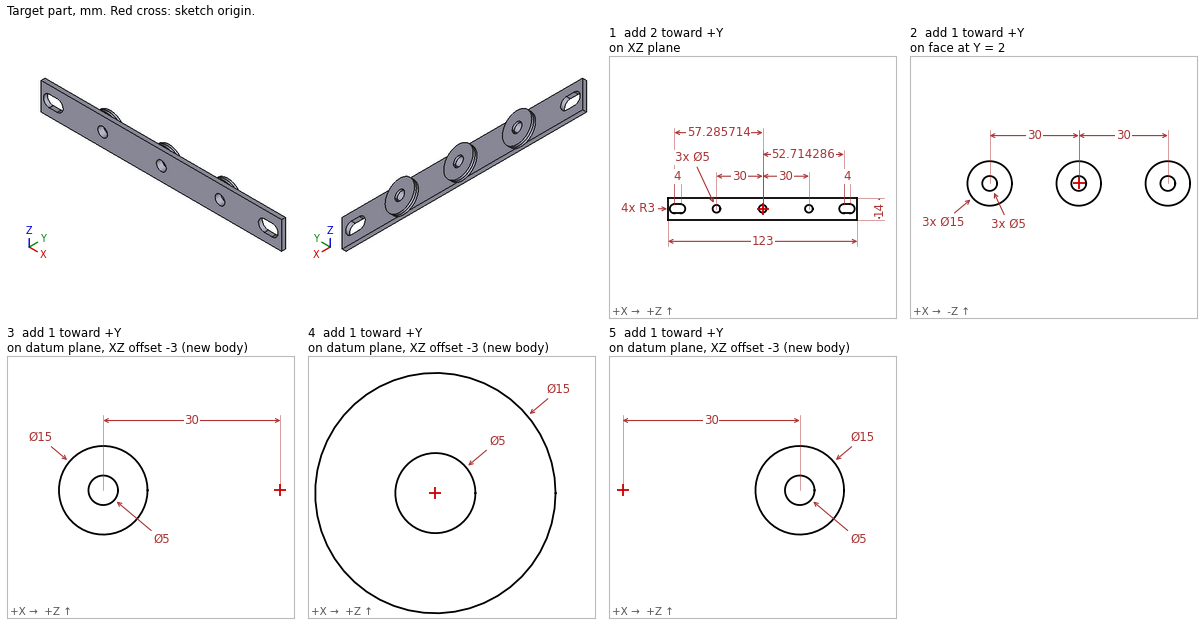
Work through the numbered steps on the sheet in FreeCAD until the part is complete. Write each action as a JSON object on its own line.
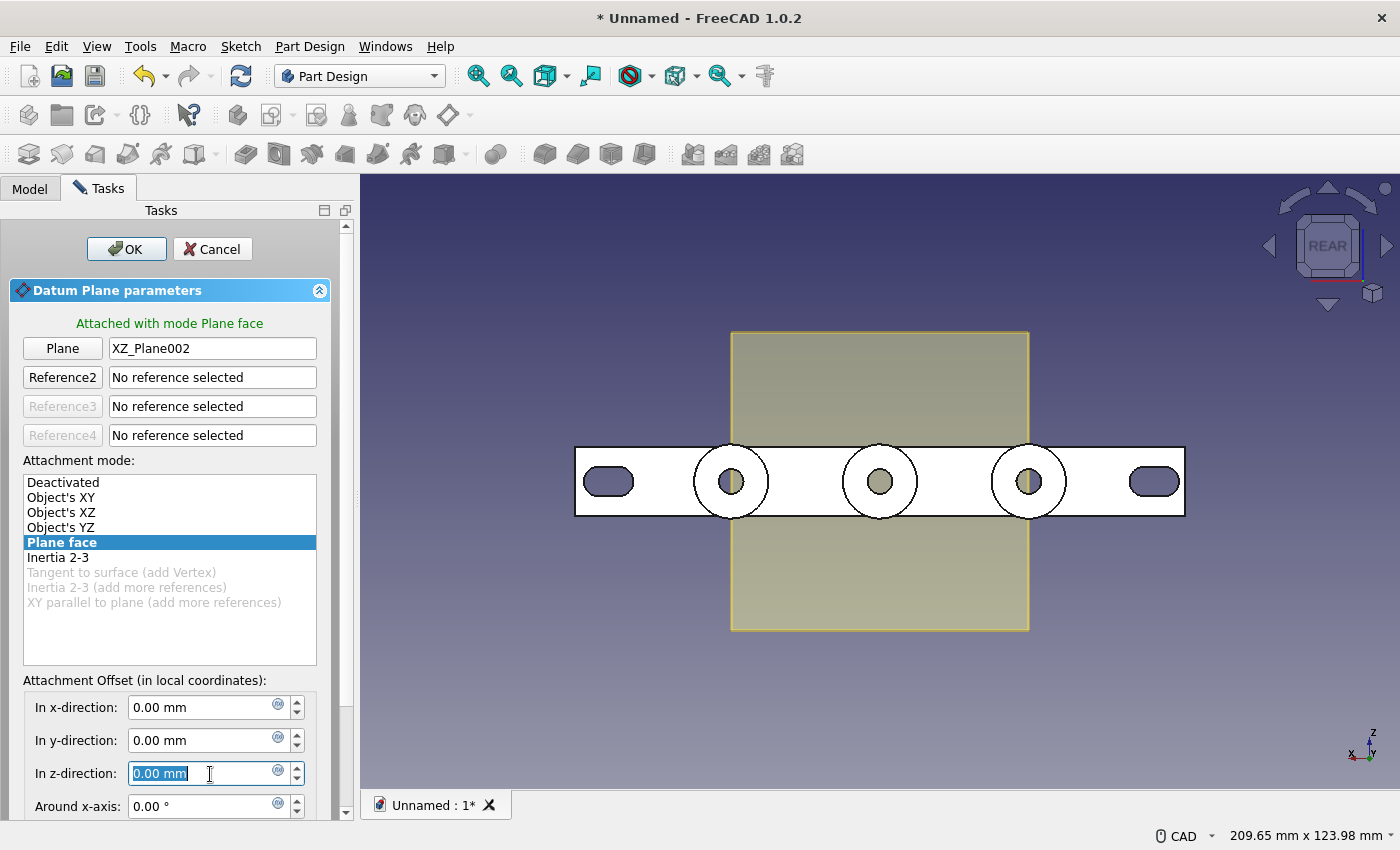
{"action": "type", "text": "-3"}
{"action": "key", "text": "Tab"}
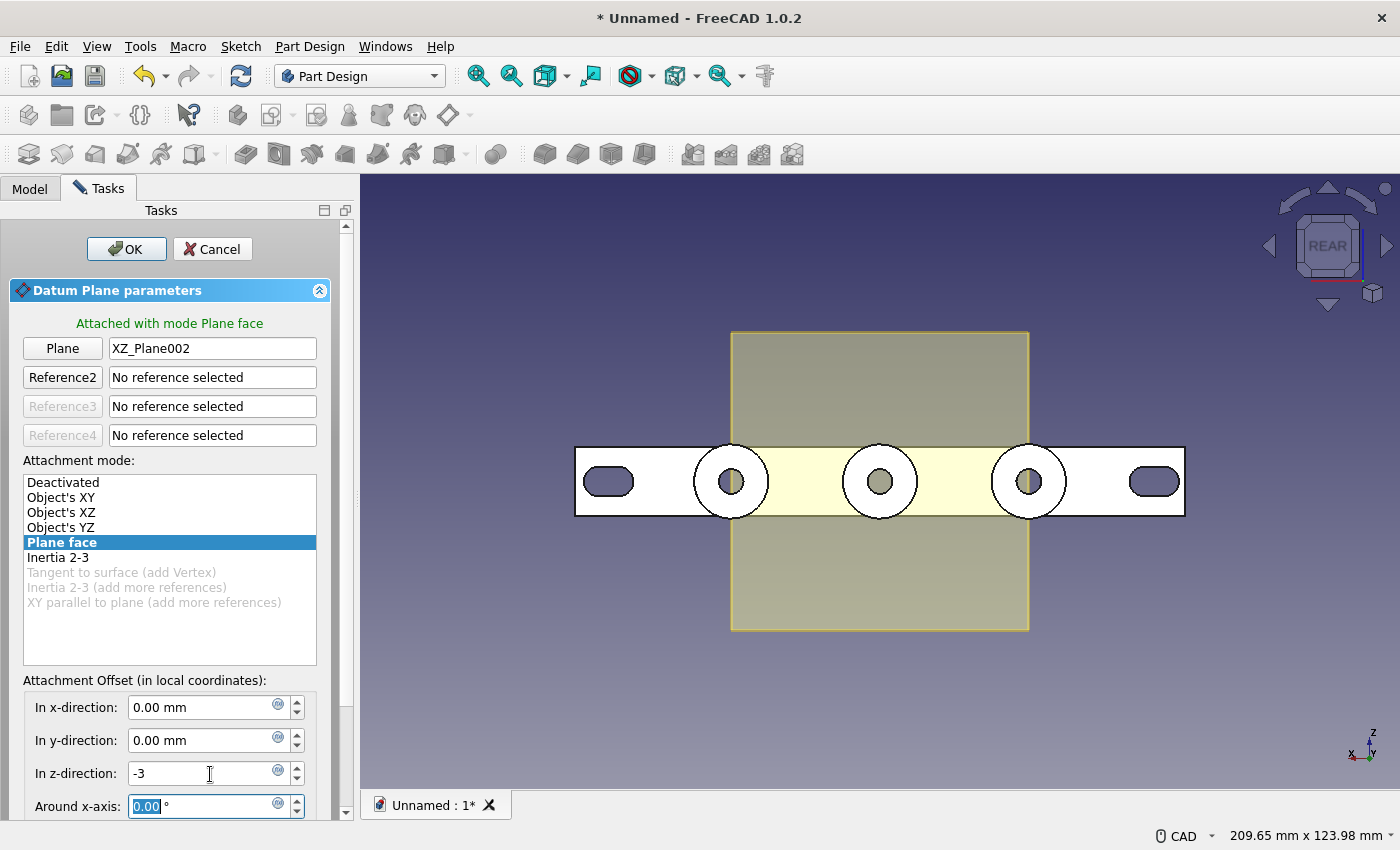
{"action": "left_click", "coordinate": [127, 249]}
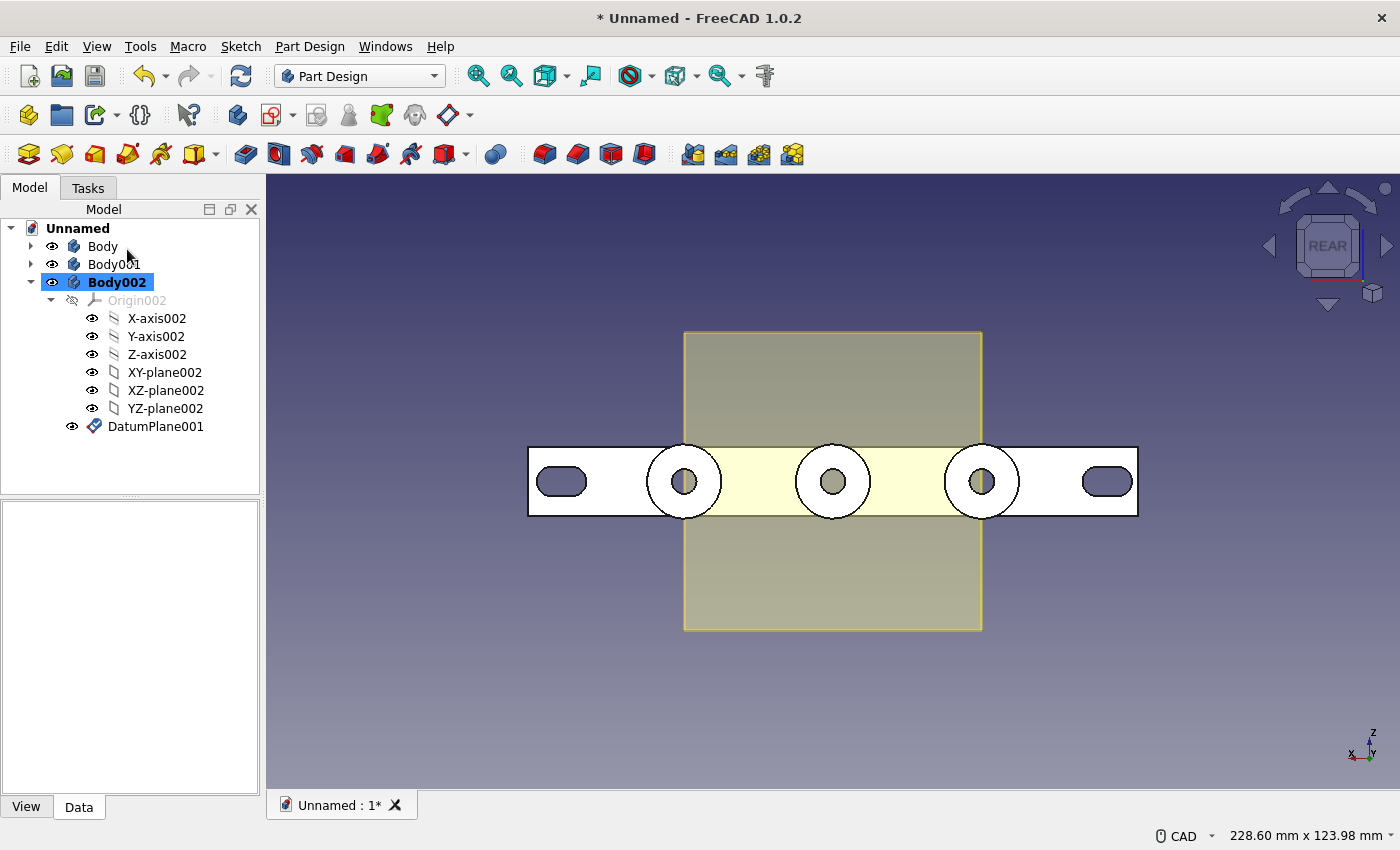
{"action": "left_click", "coordinate": [117, 426]}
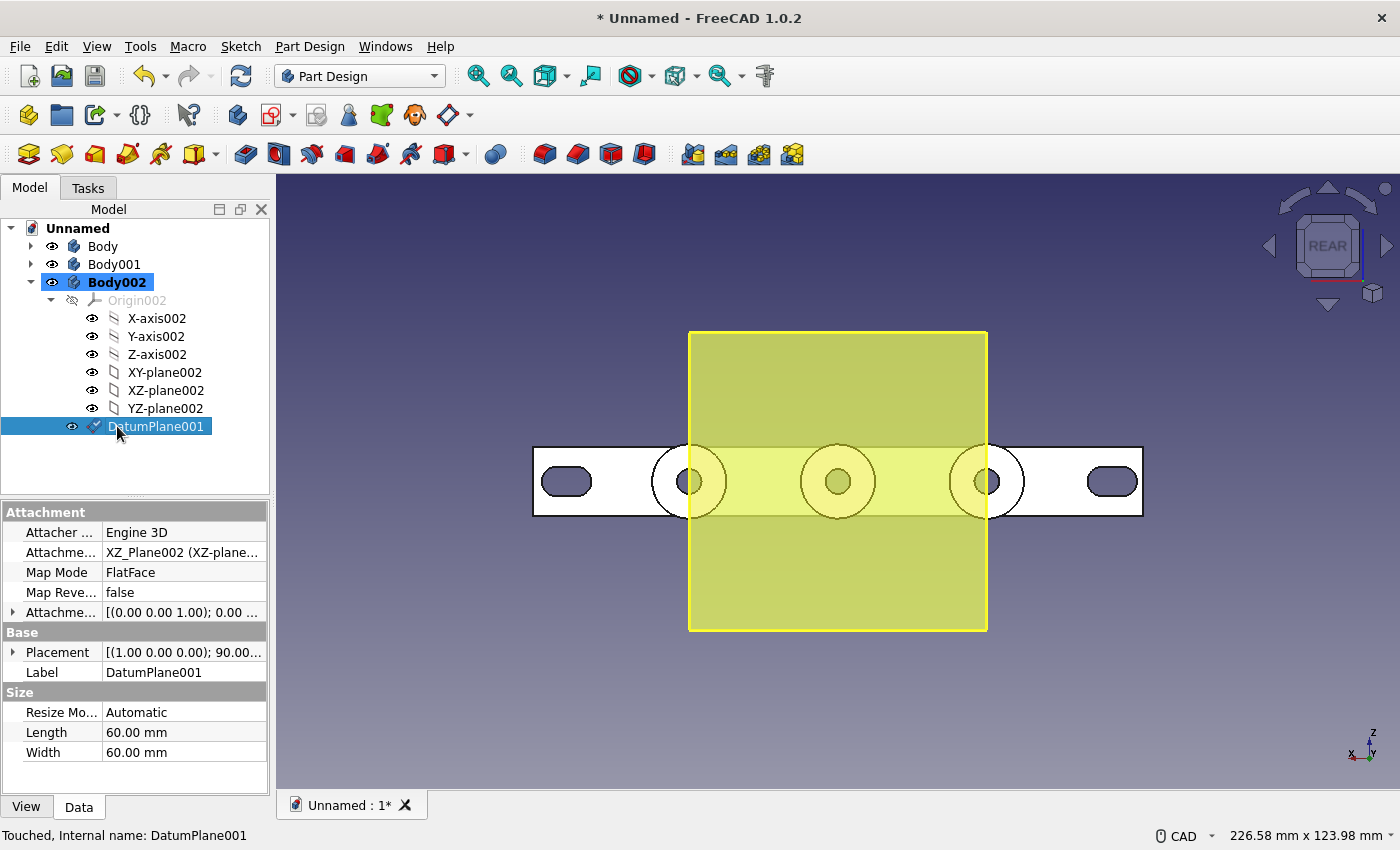
{"action": "left_click", "coordinate": [270, 116]}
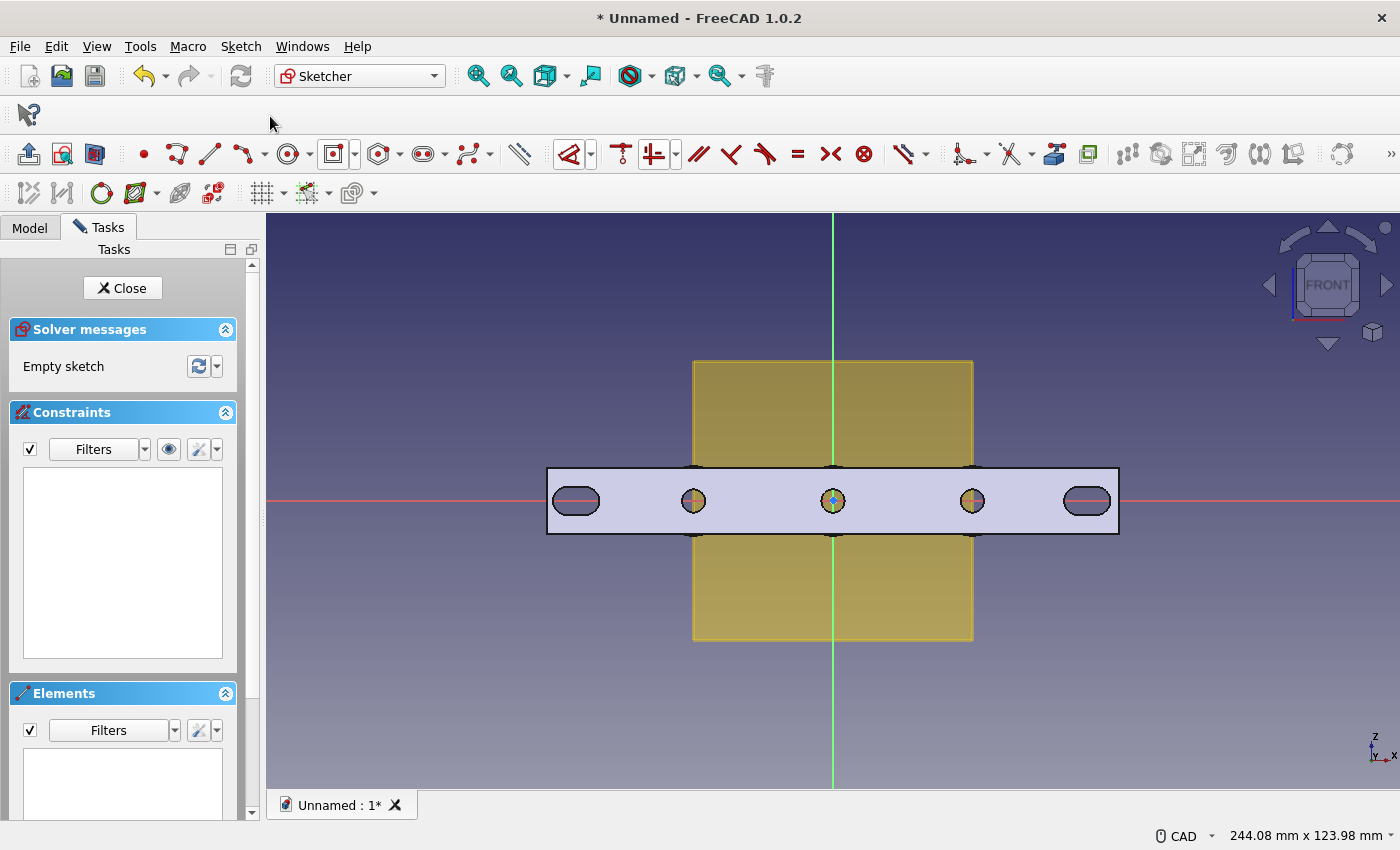
{"action": "scroll", "coordinate": [850, 501], "scroll_direction": "up", "scroll_amount": 8}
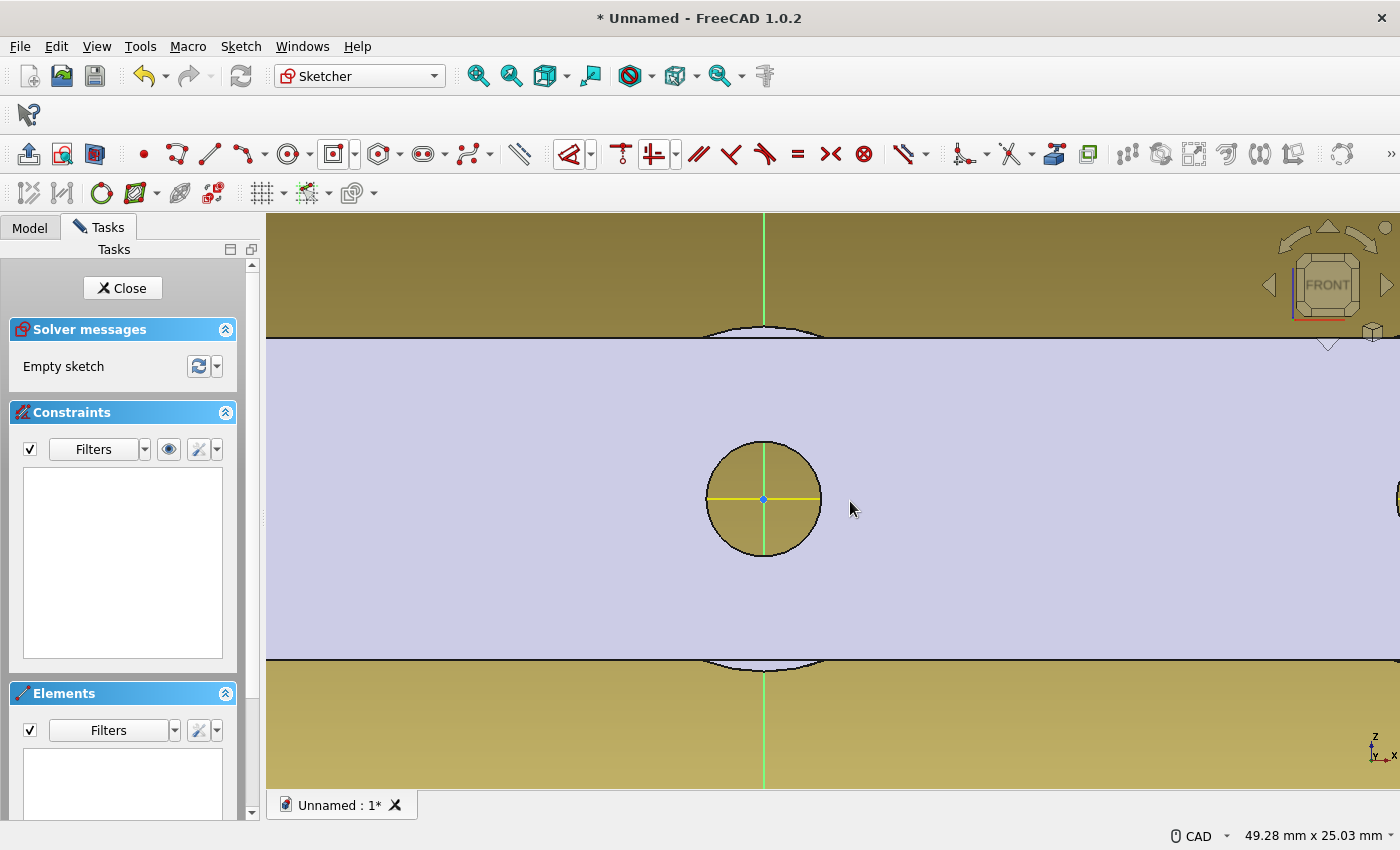
{"action": "left_click", "coordinate": [288, 154]}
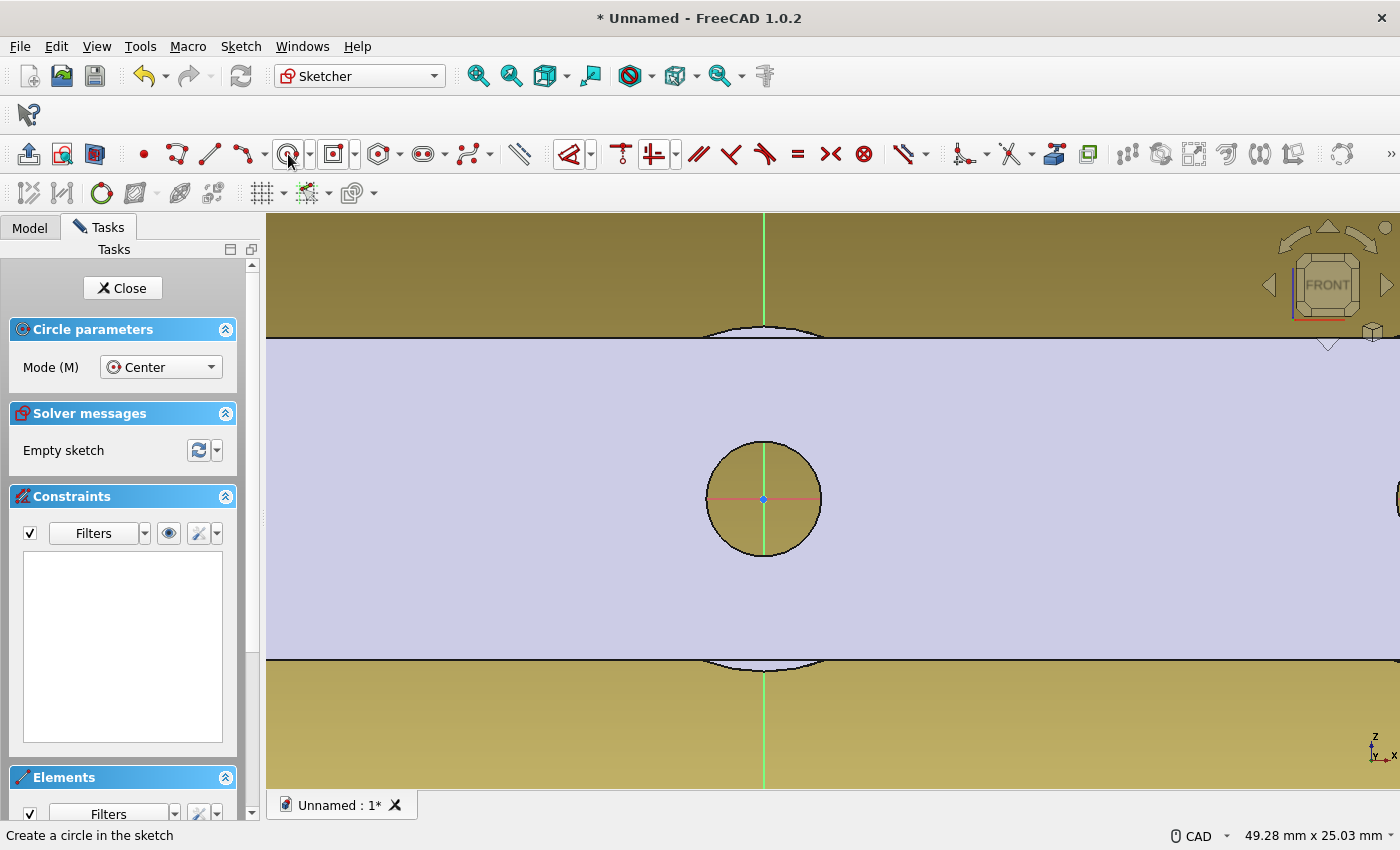
{"action": "left_click", "coordinate": [764, 499]}
{"action": "left_click", "coordinate": [886, 377]}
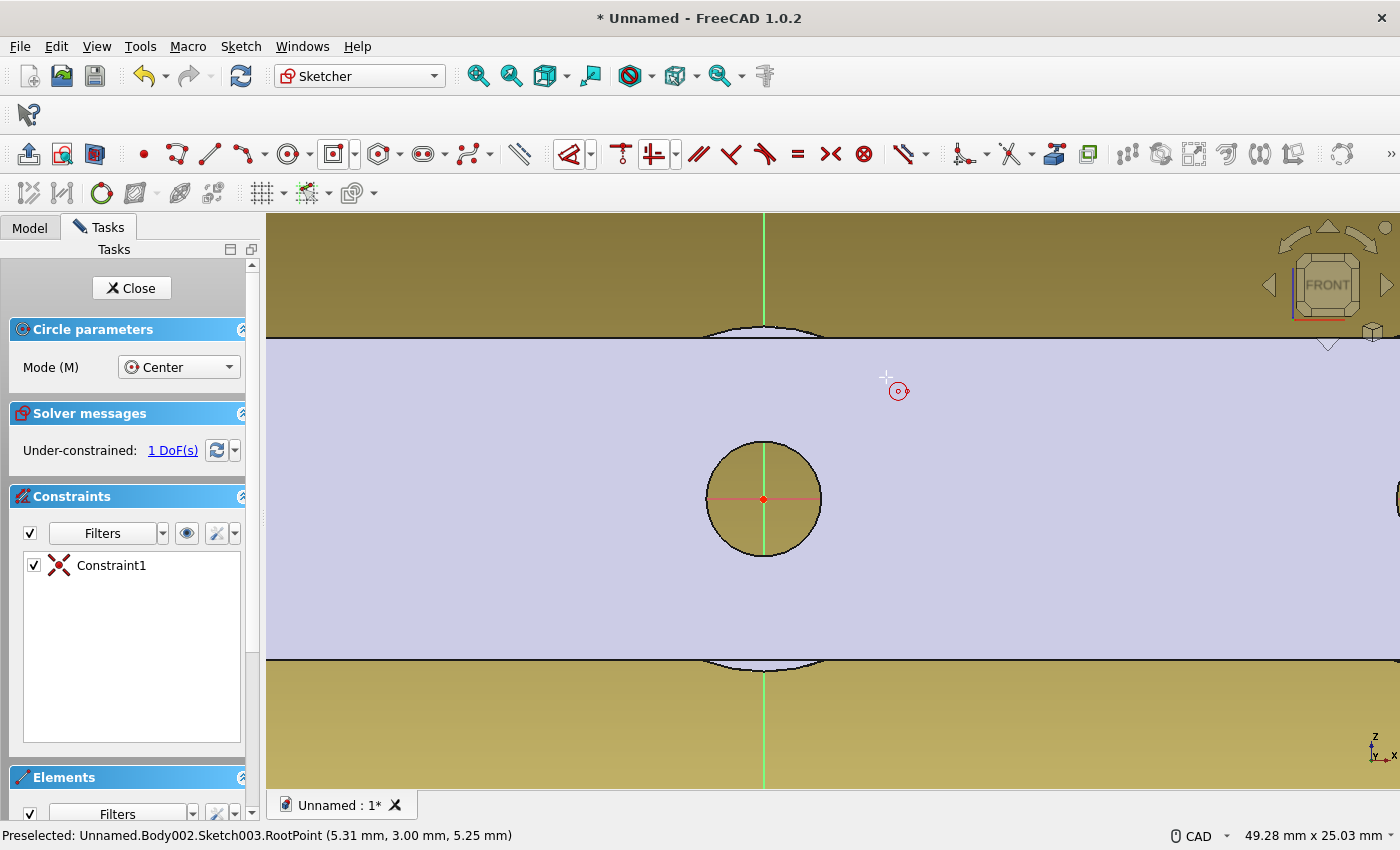
{"action": "left_click", "coordinate": [764, 499]}
{"action": "left_click", "coordinate": [804, 458]}
{"action": "key", "text": "Escape"}